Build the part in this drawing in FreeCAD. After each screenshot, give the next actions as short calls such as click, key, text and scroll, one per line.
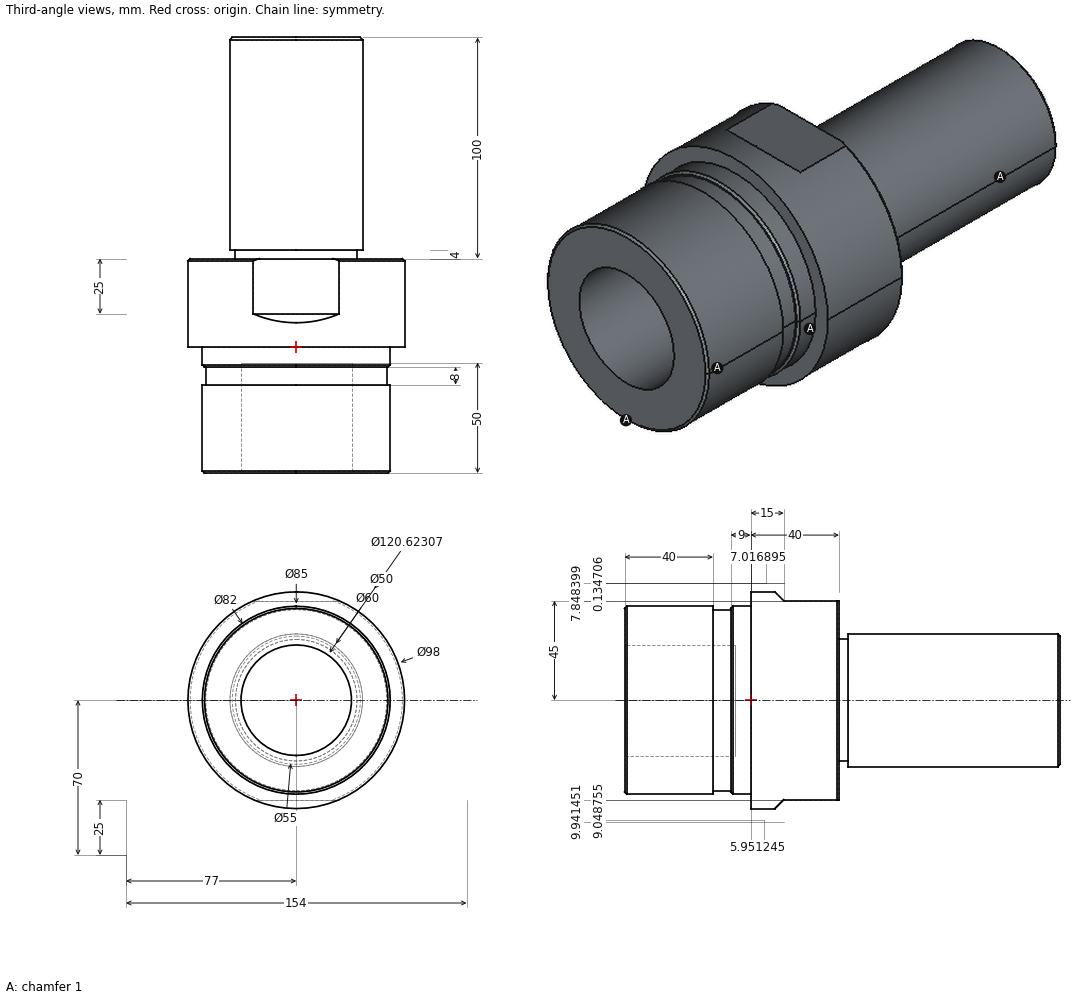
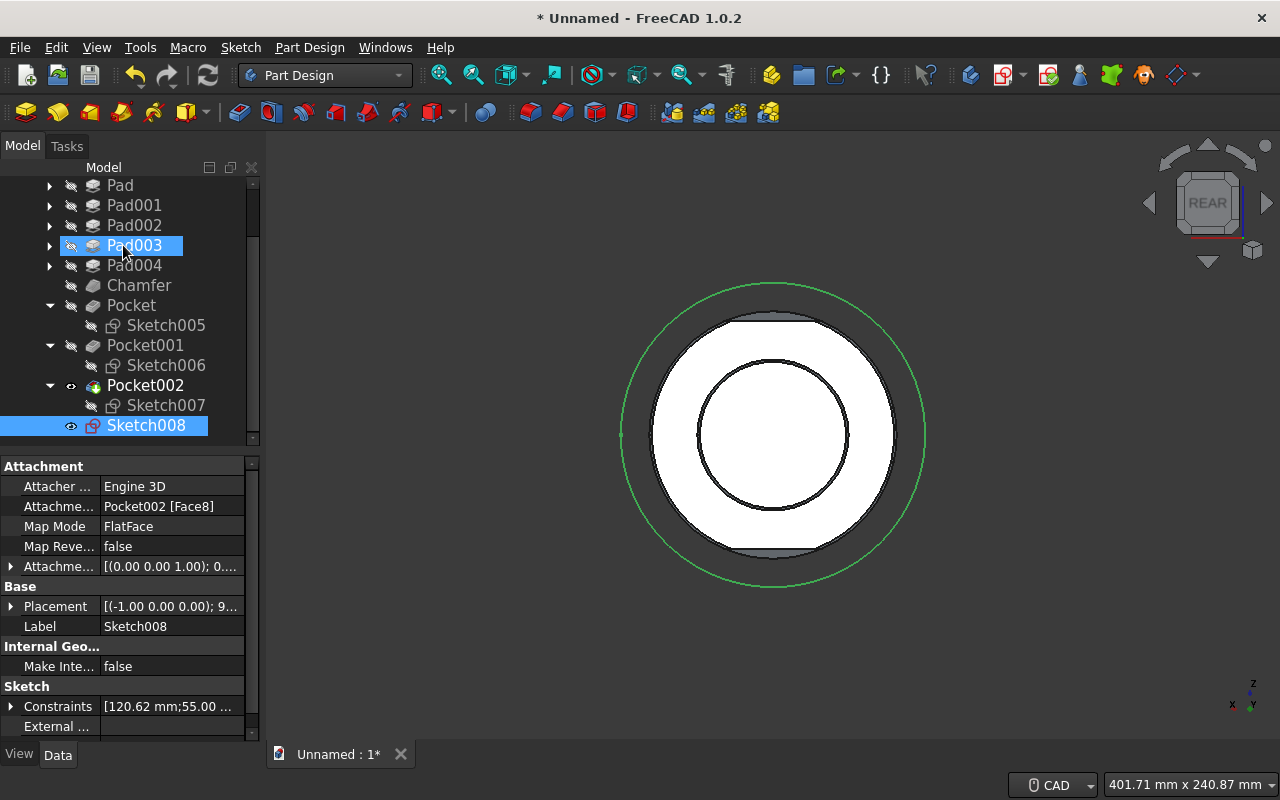
click(240, 112)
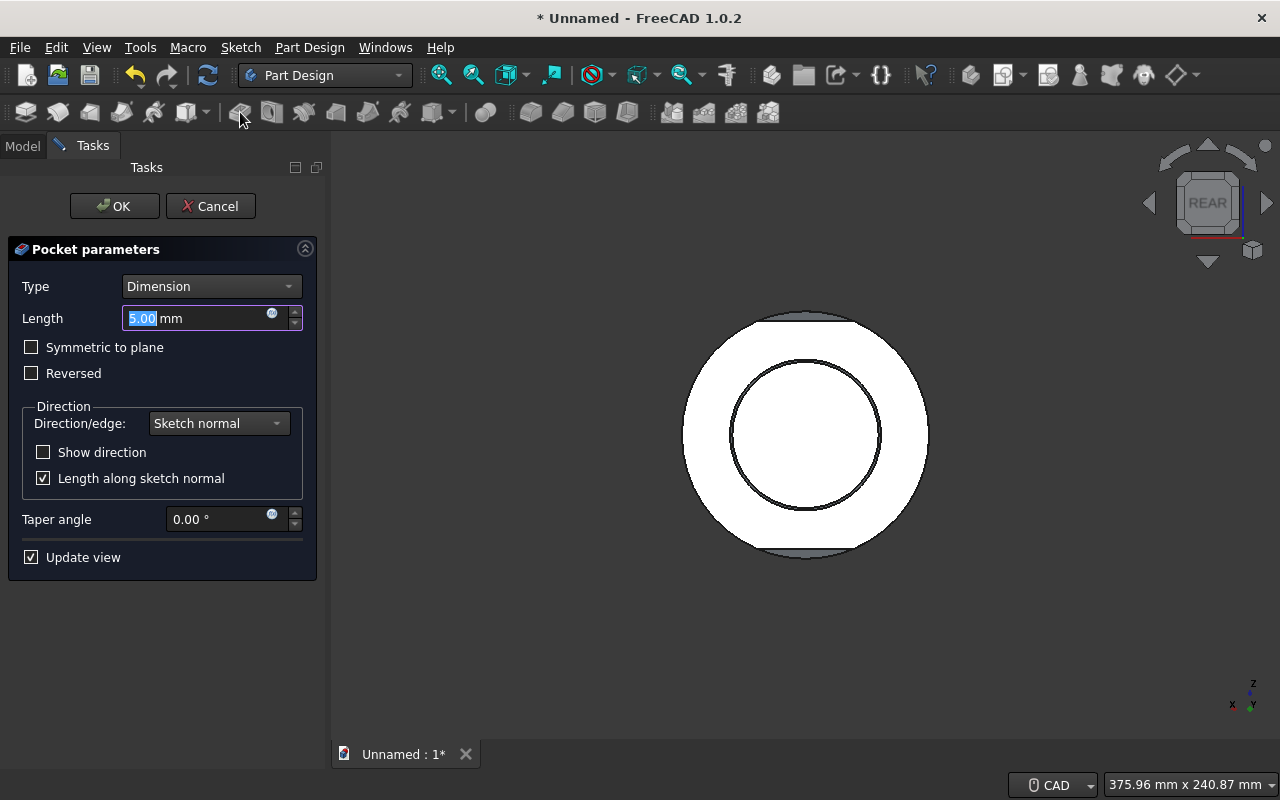
text(4)
key(Tab)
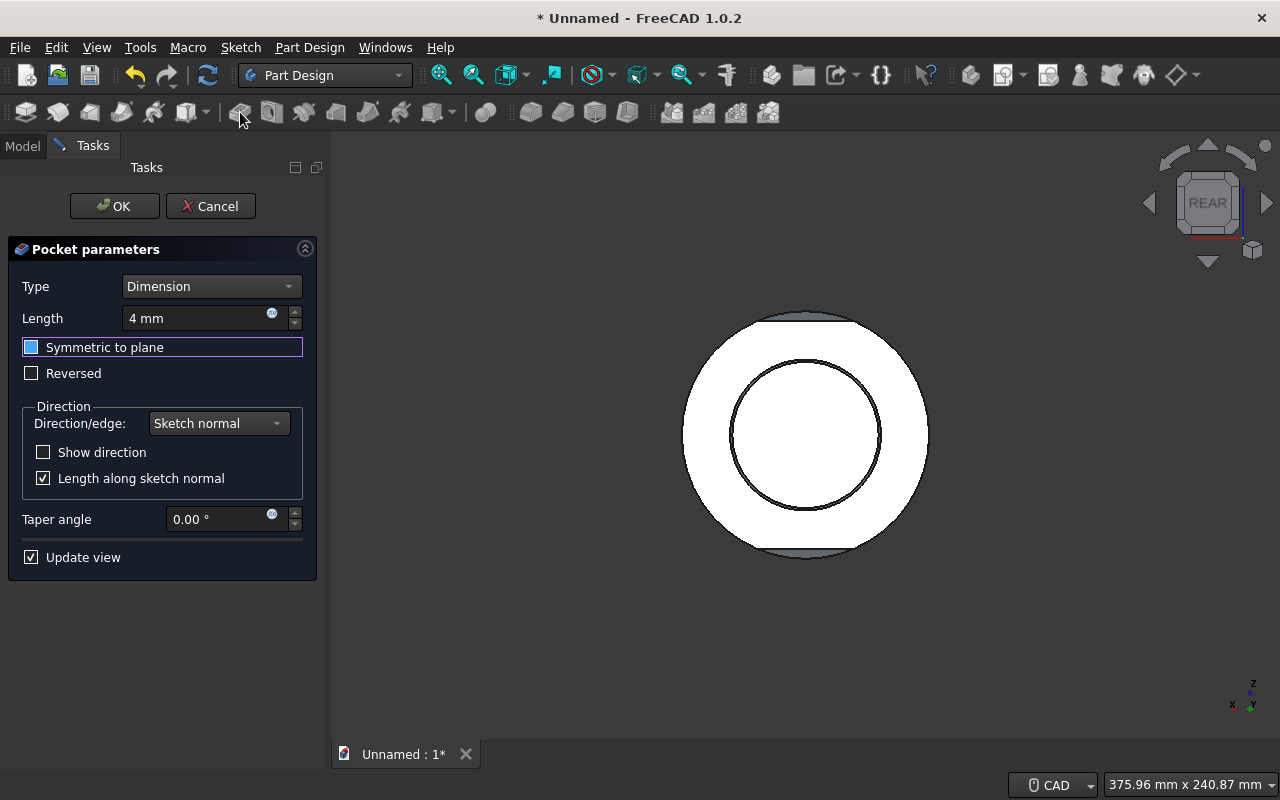
click(30, 373)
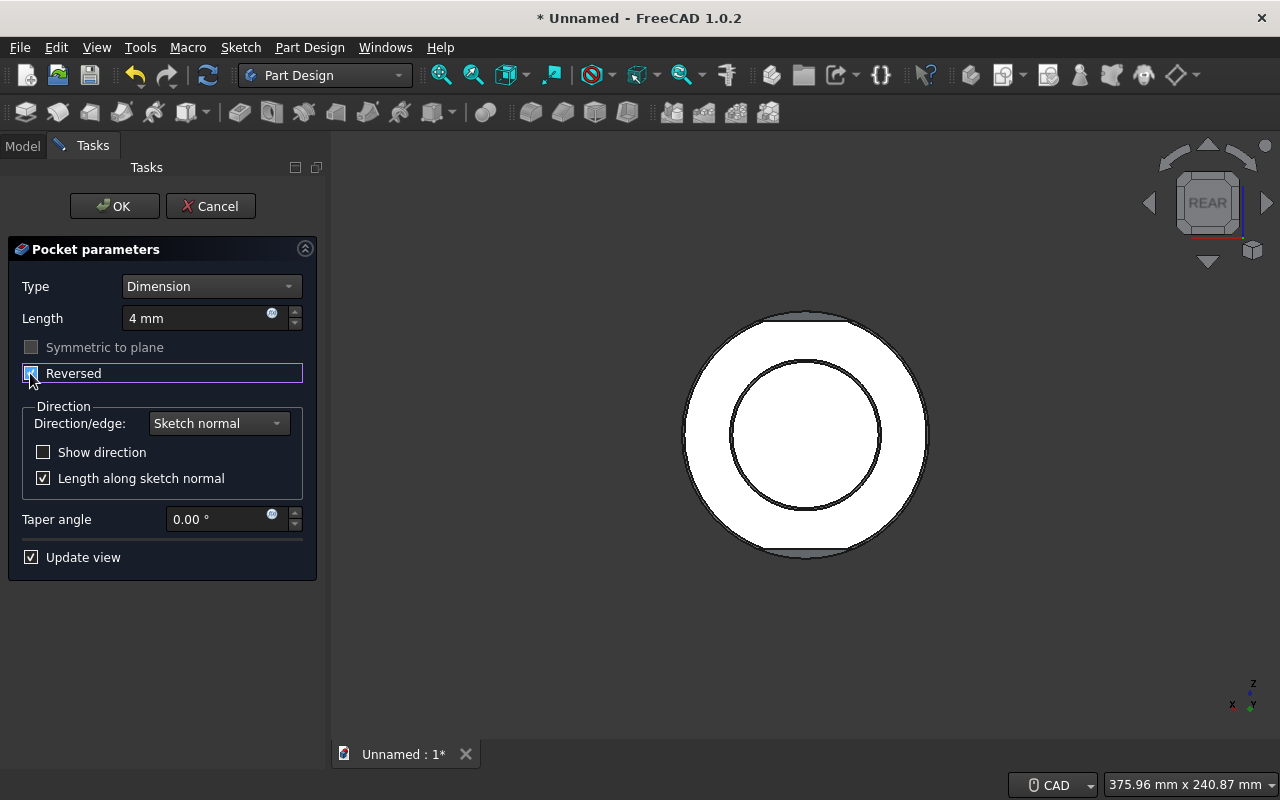
click(115, 206)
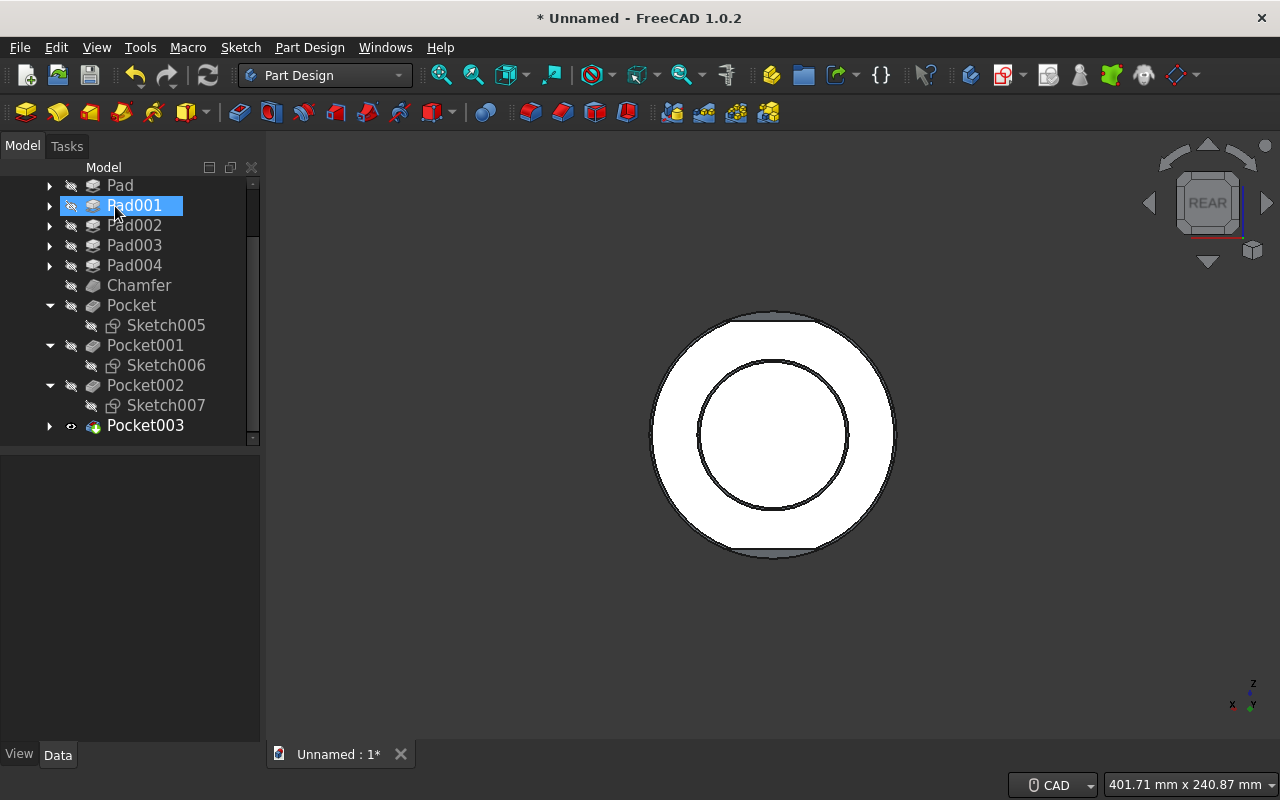
click(442, 76)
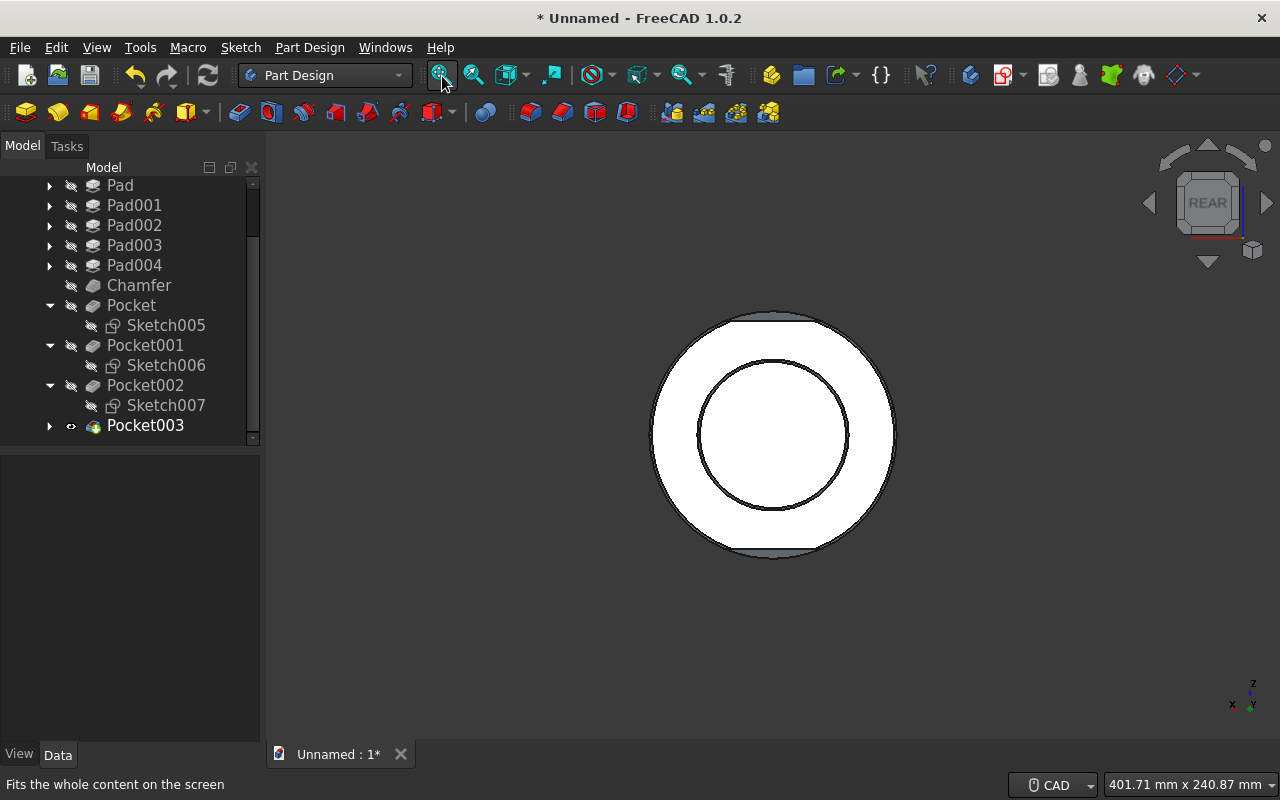
key(0)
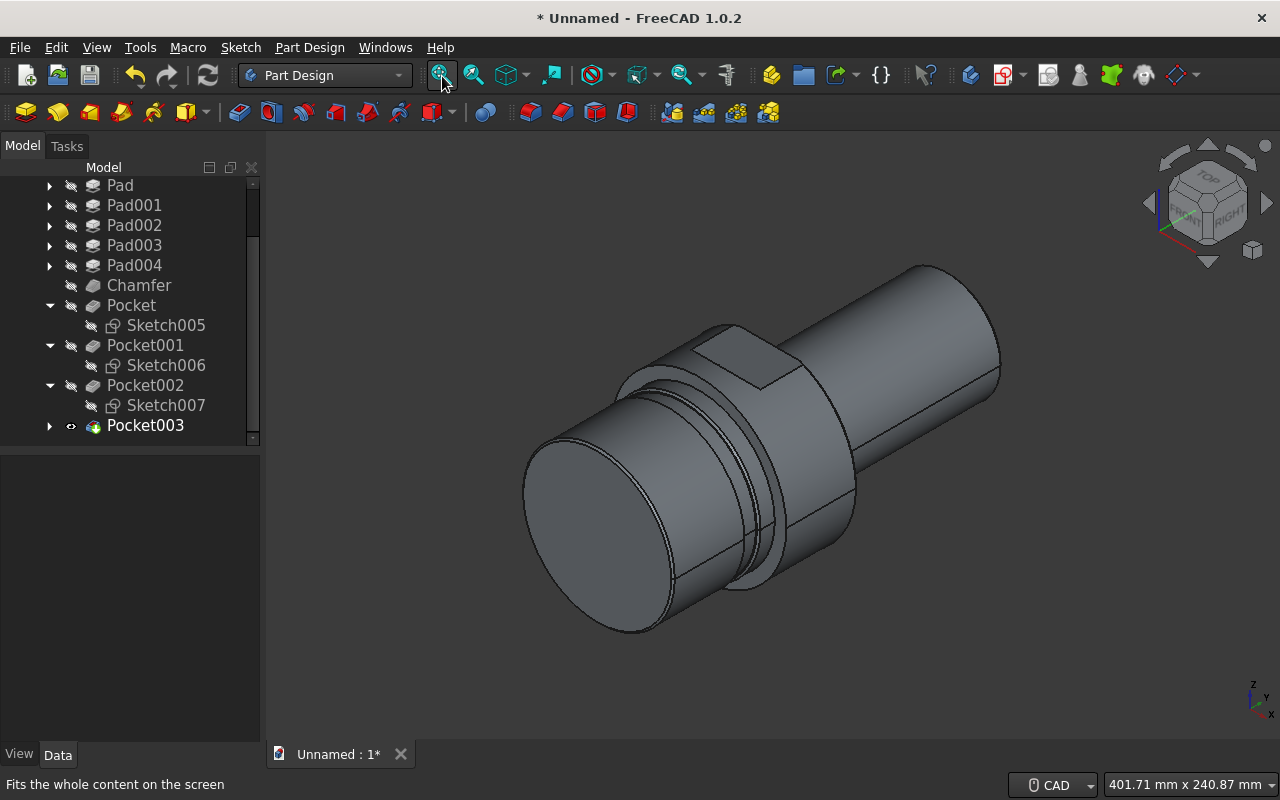
click(597, 536)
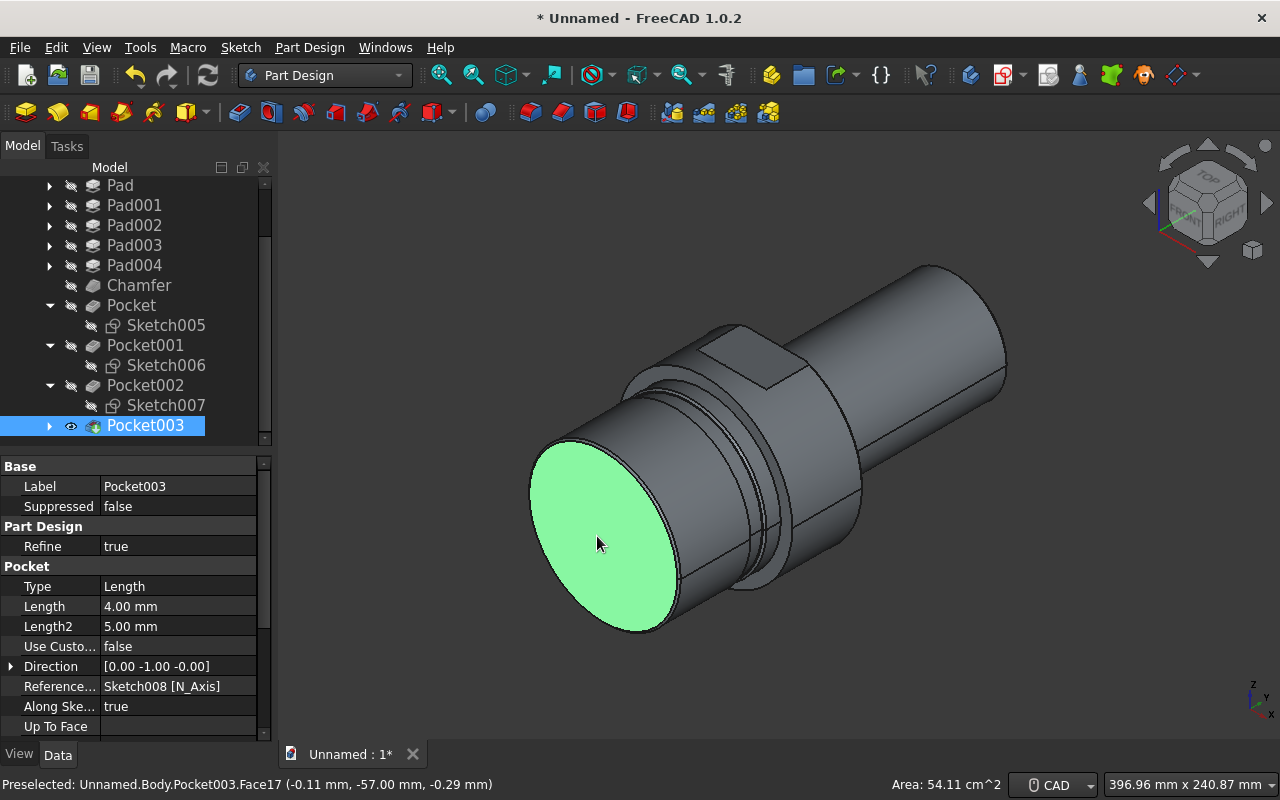
click(1004, 76)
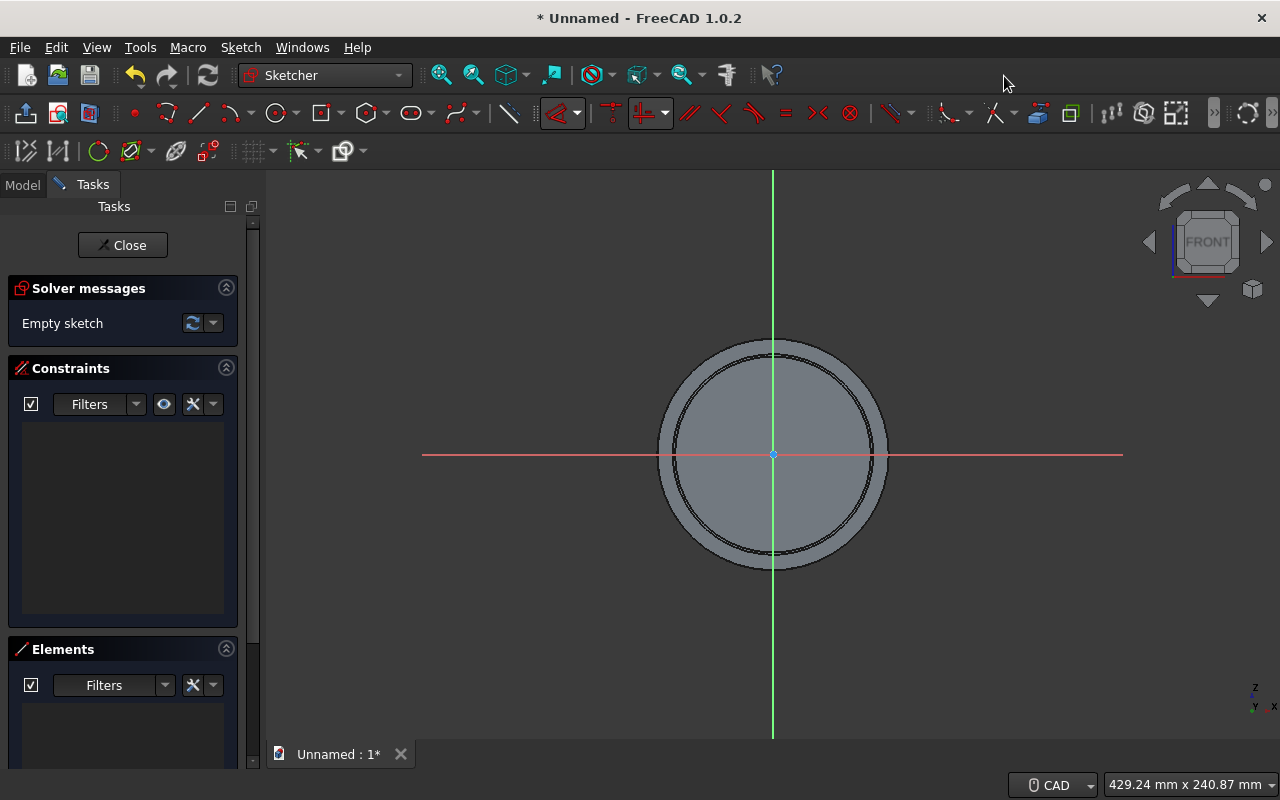
scroll(803, 455, up, 6)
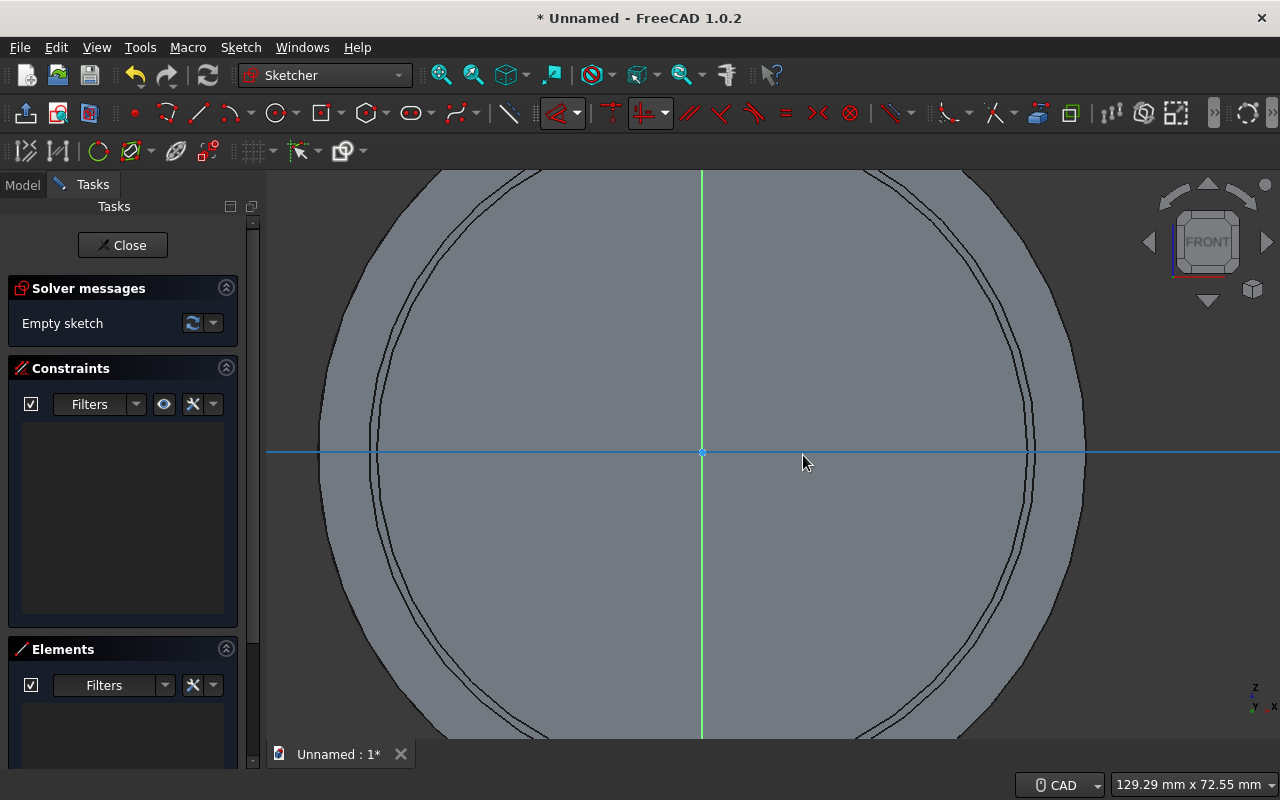
click(276, 114)